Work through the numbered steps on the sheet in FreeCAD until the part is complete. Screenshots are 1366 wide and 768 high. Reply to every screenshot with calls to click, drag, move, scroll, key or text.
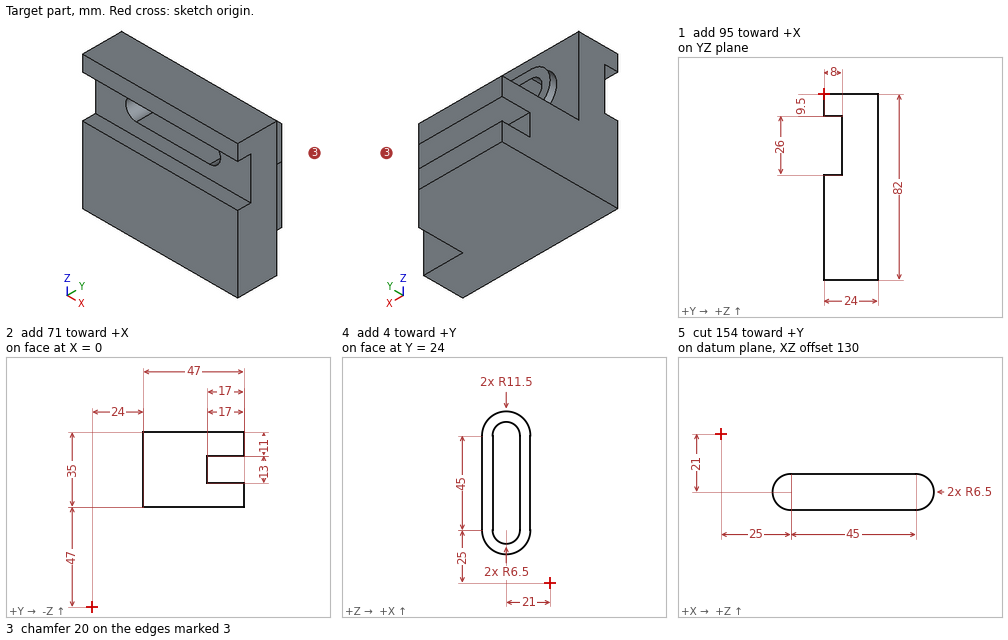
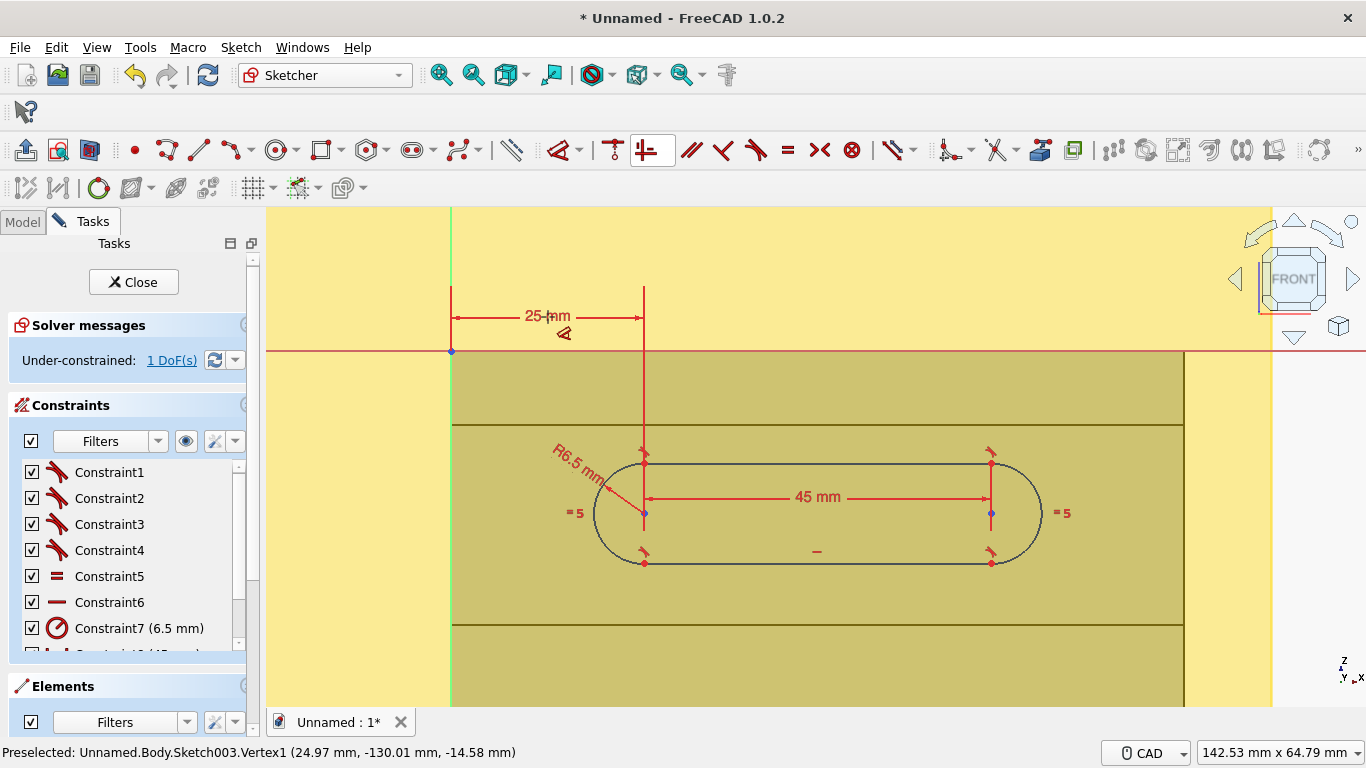
click(644, 514)
click(417, 433)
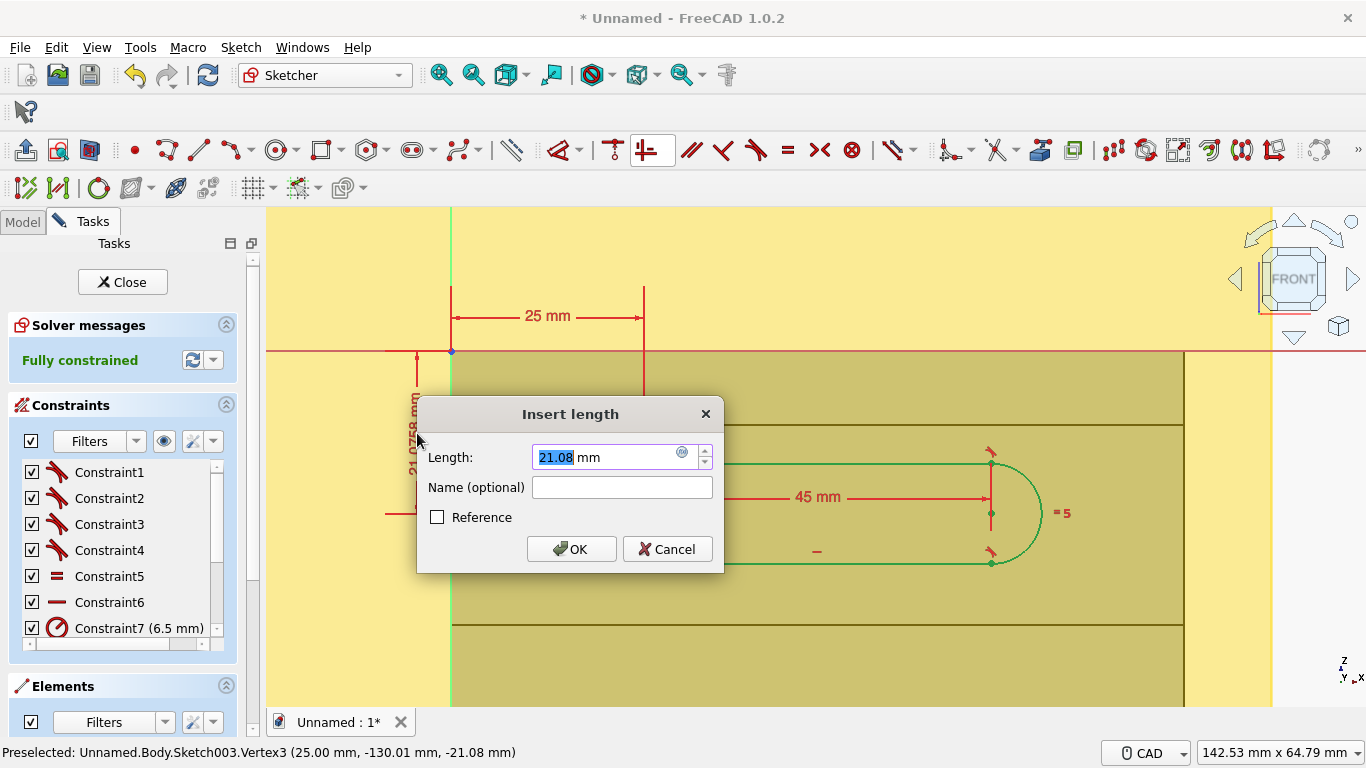
text(21)
key(Return)
key(Escape)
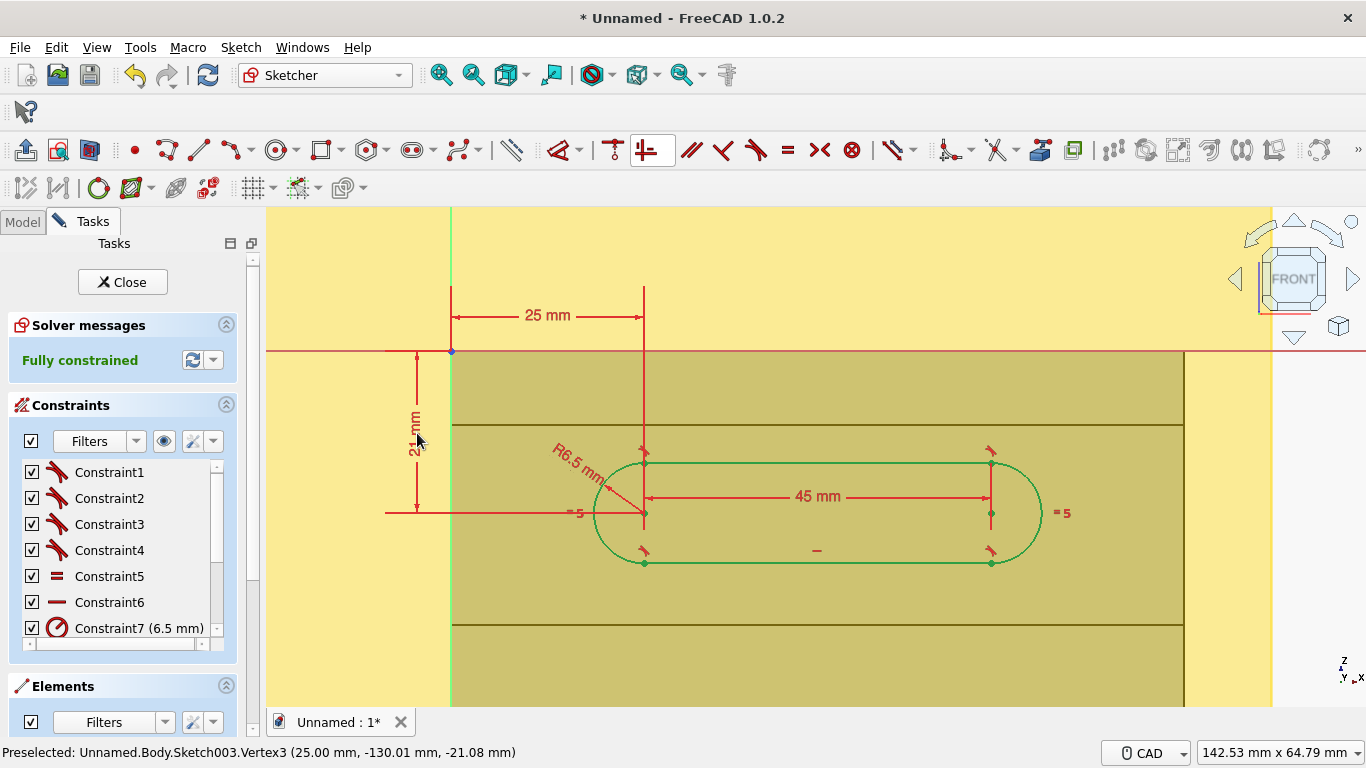
click(123, 282)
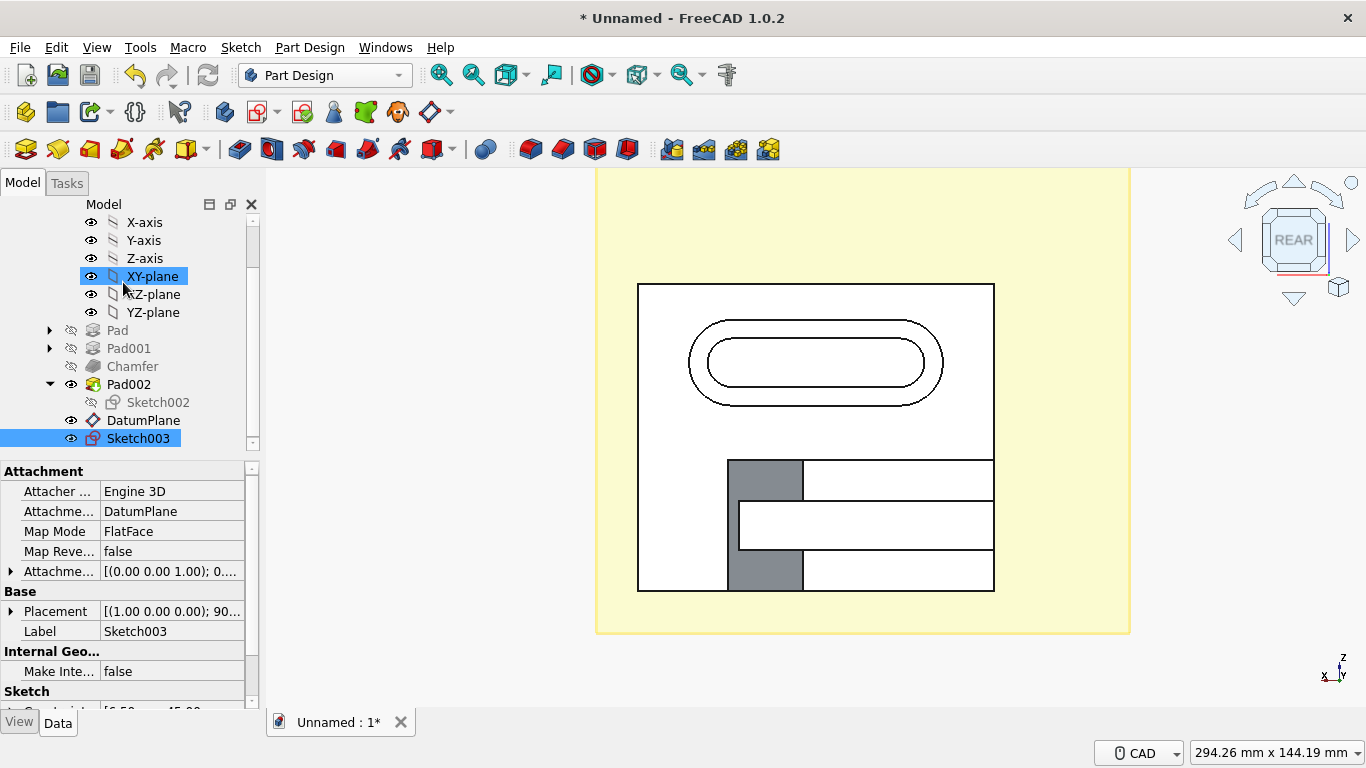
click(240, 150)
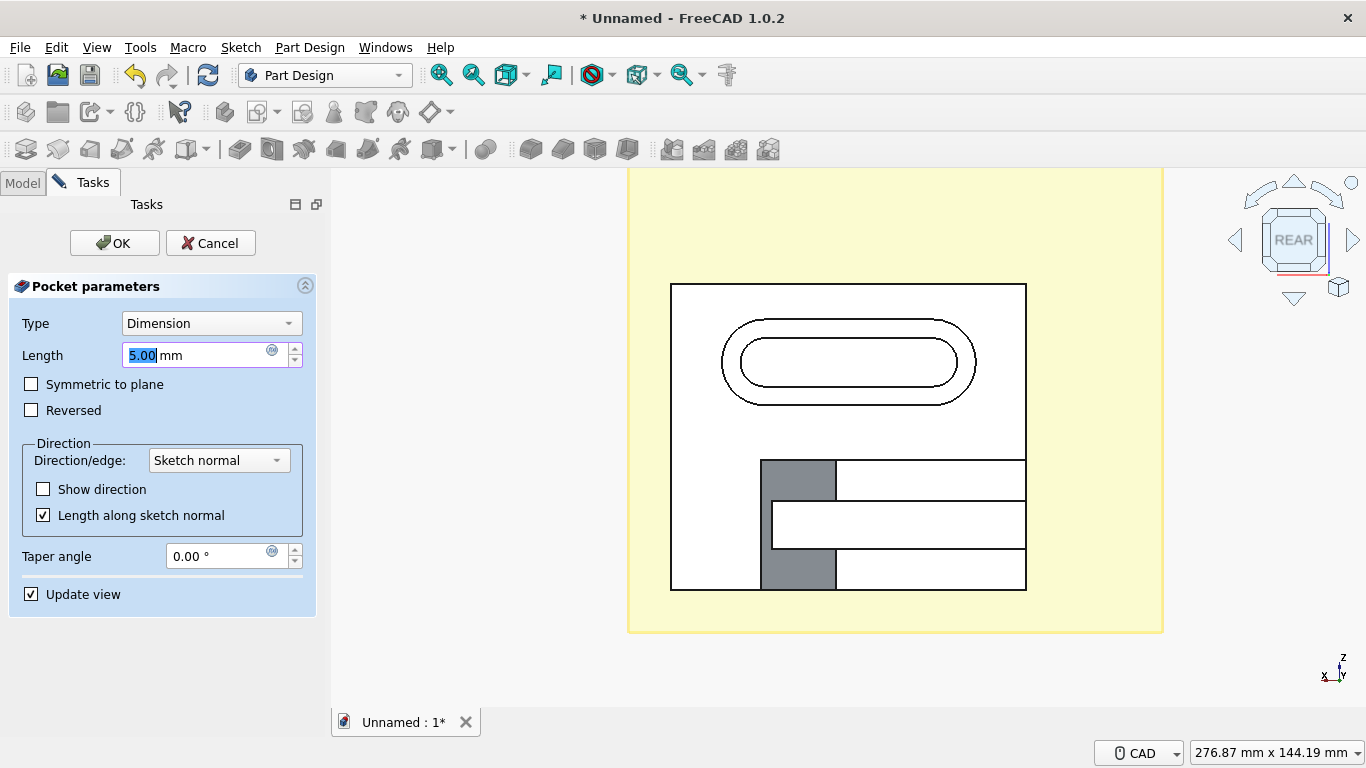
text(154)
key(Tab)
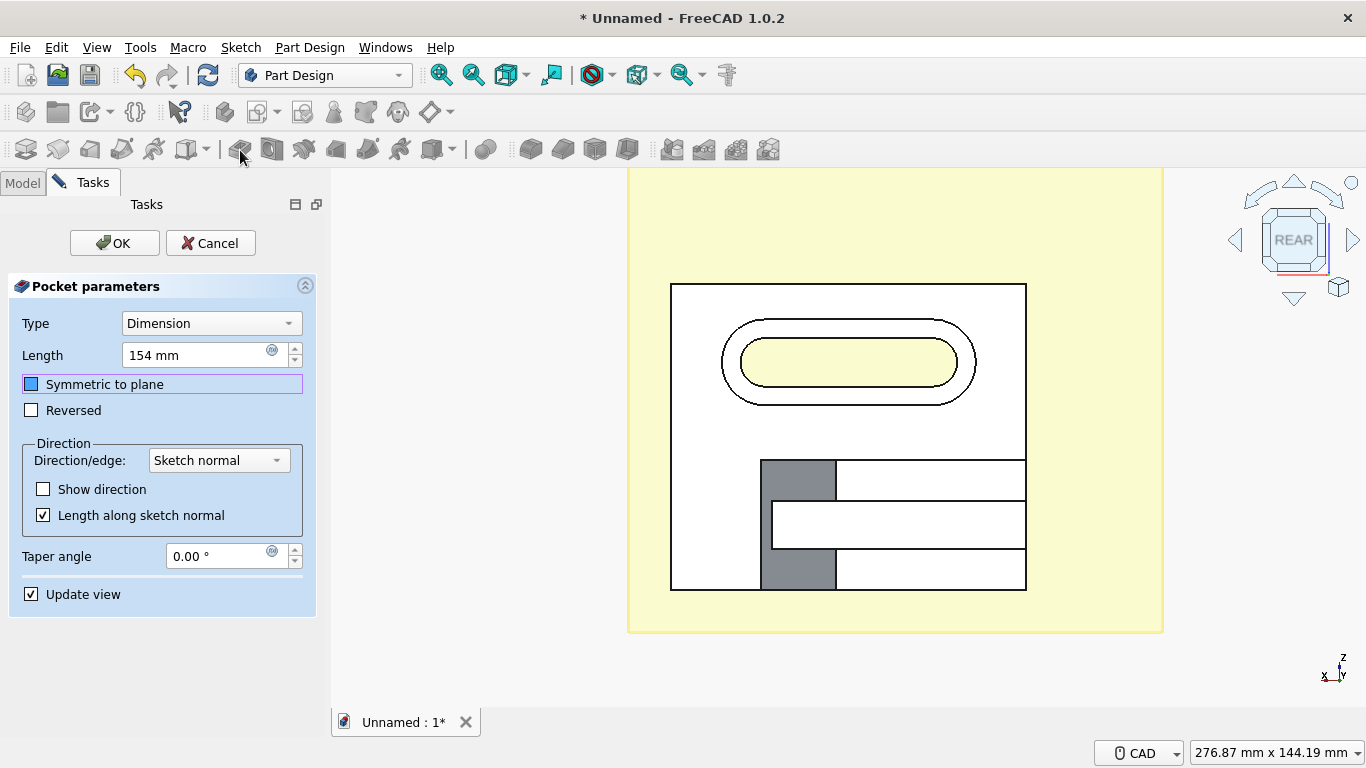
click(115, 243)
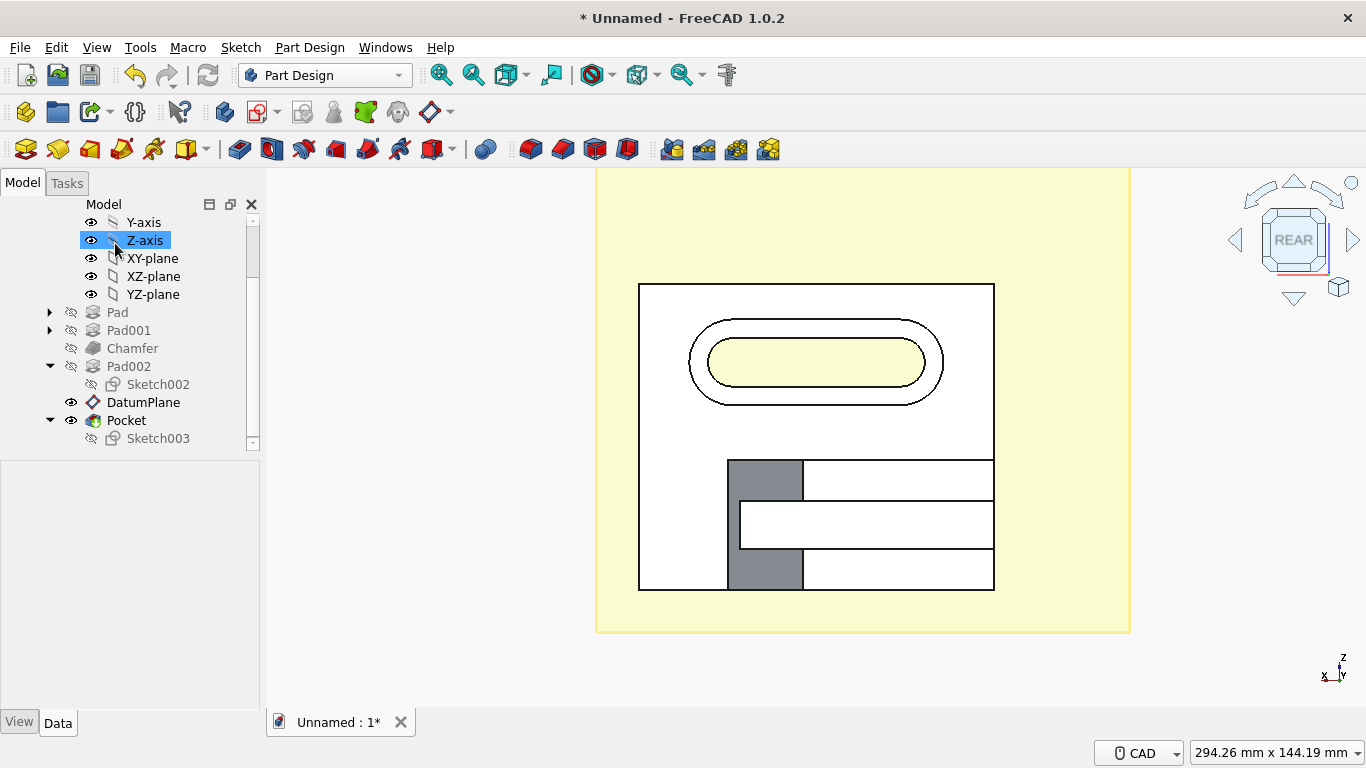
click(116, 402)
key(space)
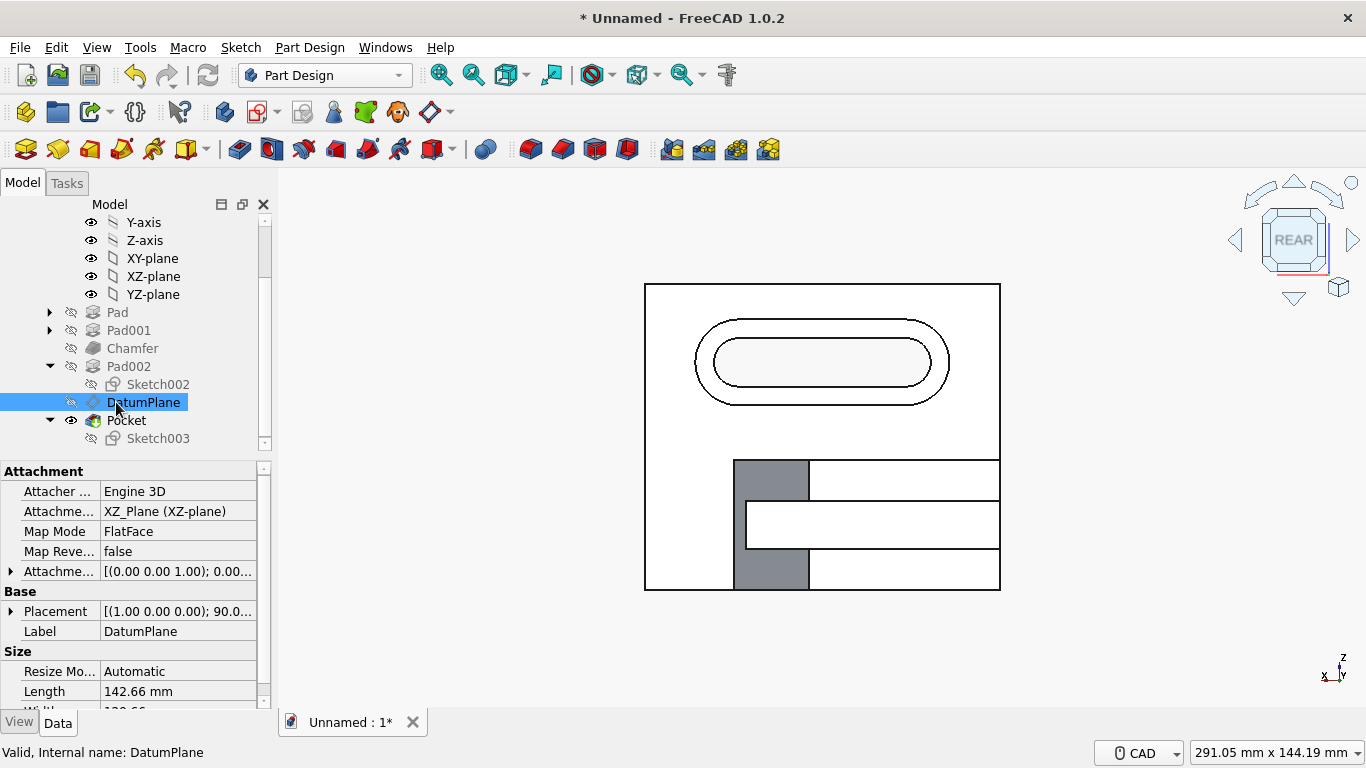
key(0)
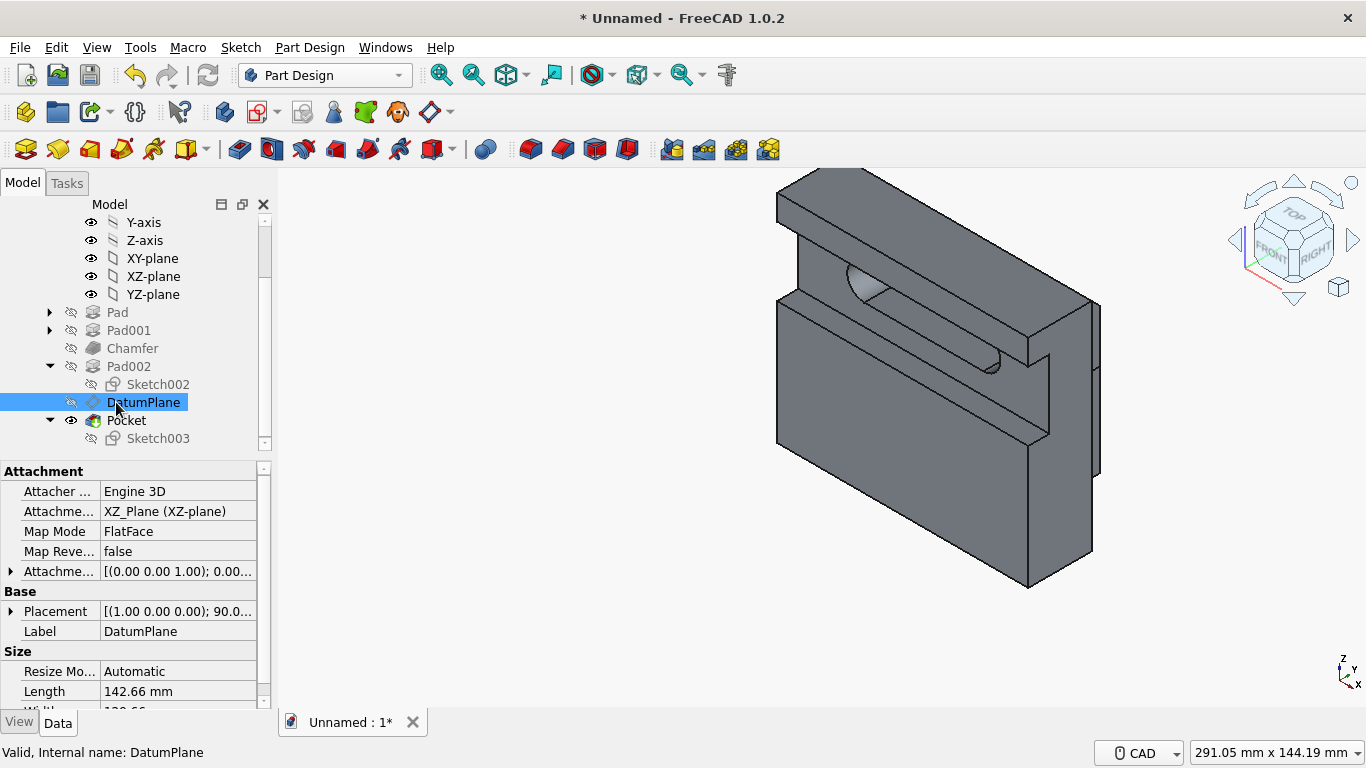
click(442, 76)